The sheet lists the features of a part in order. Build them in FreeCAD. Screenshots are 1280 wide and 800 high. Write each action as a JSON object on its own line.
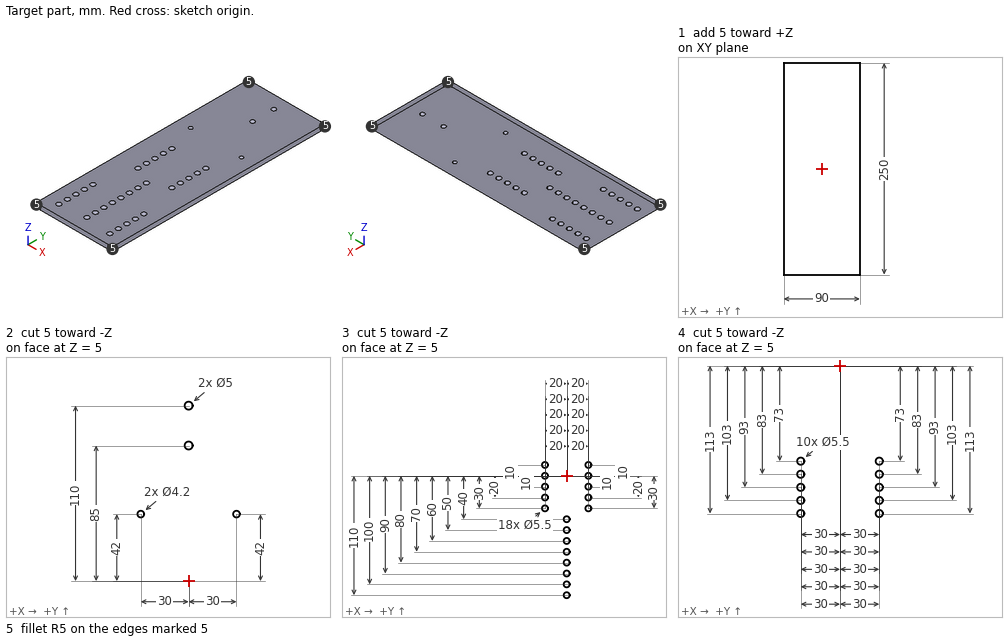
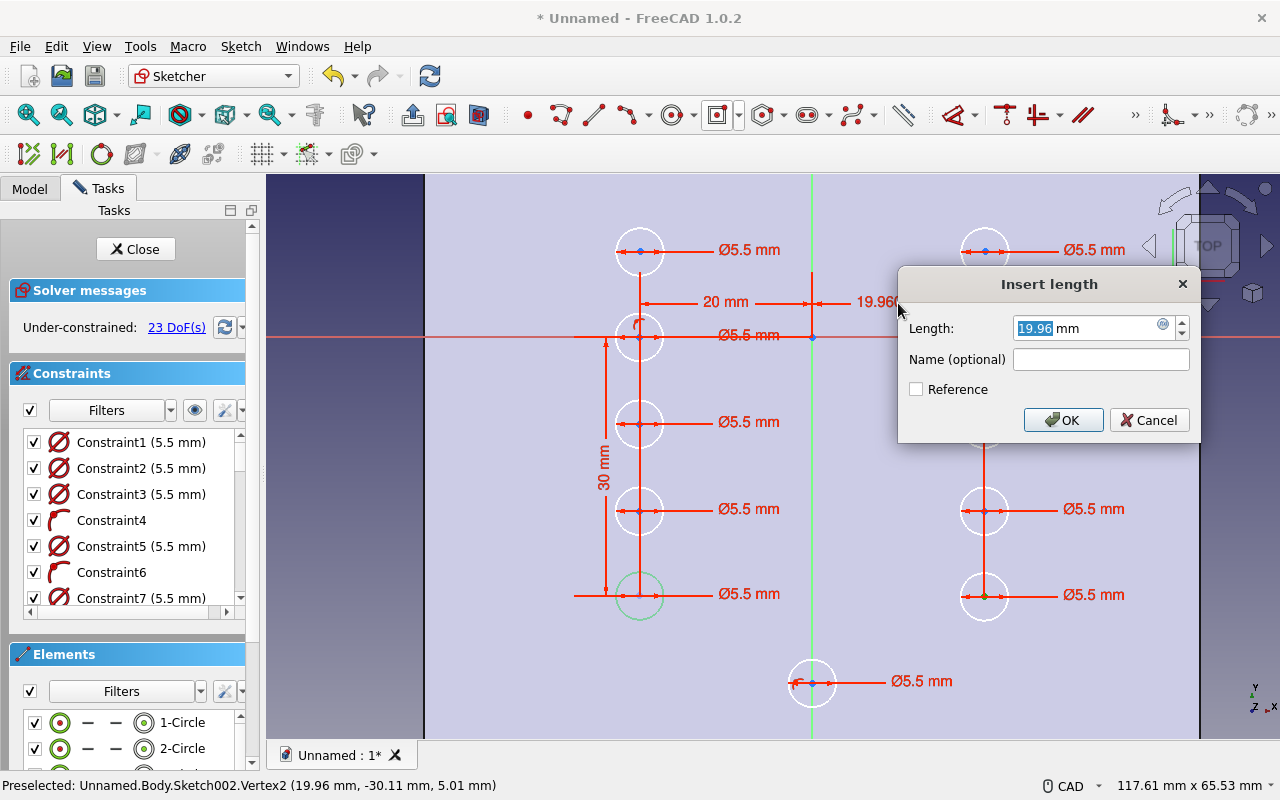
{"action": "type", "text": "20"}
{"action": "key", "text": "Return"}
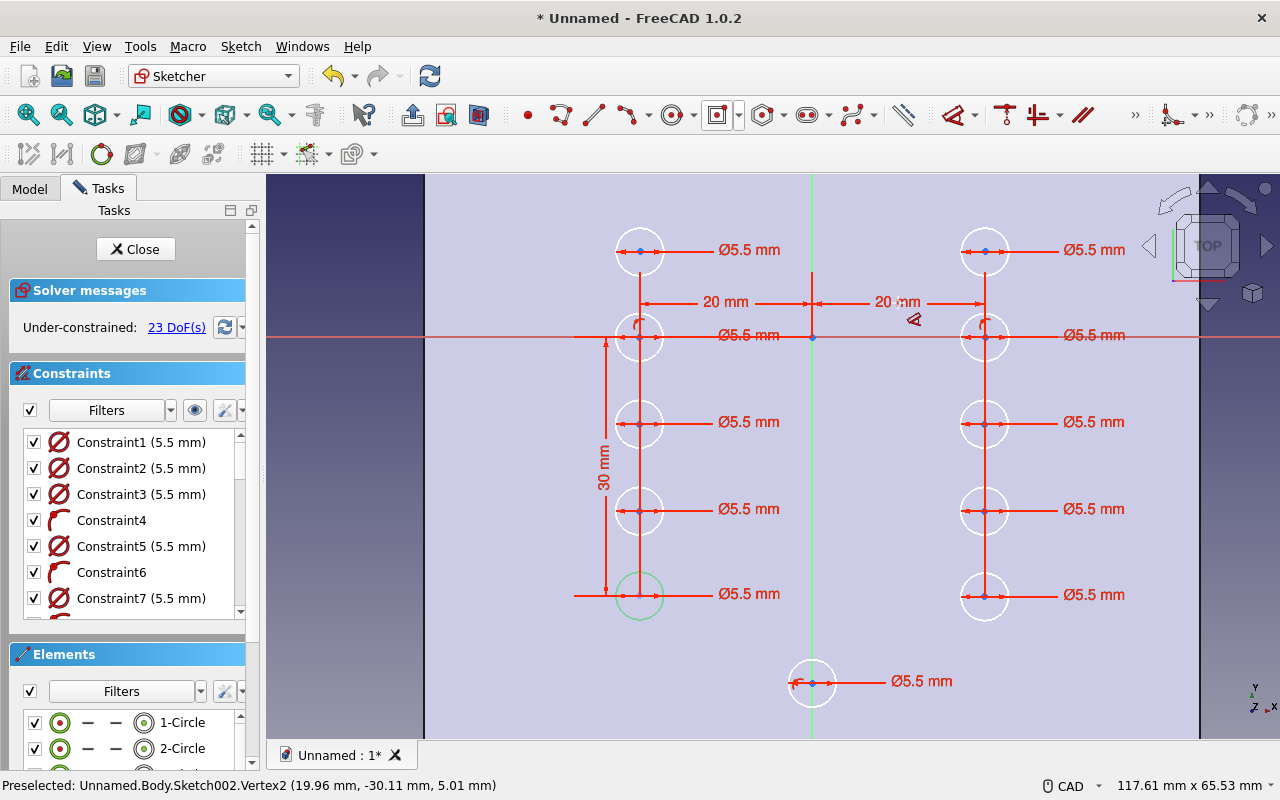
{"action": "left_click", "coordinate": [985, 597]}
{"action": "left_click", "coordinate": [1019, 467]}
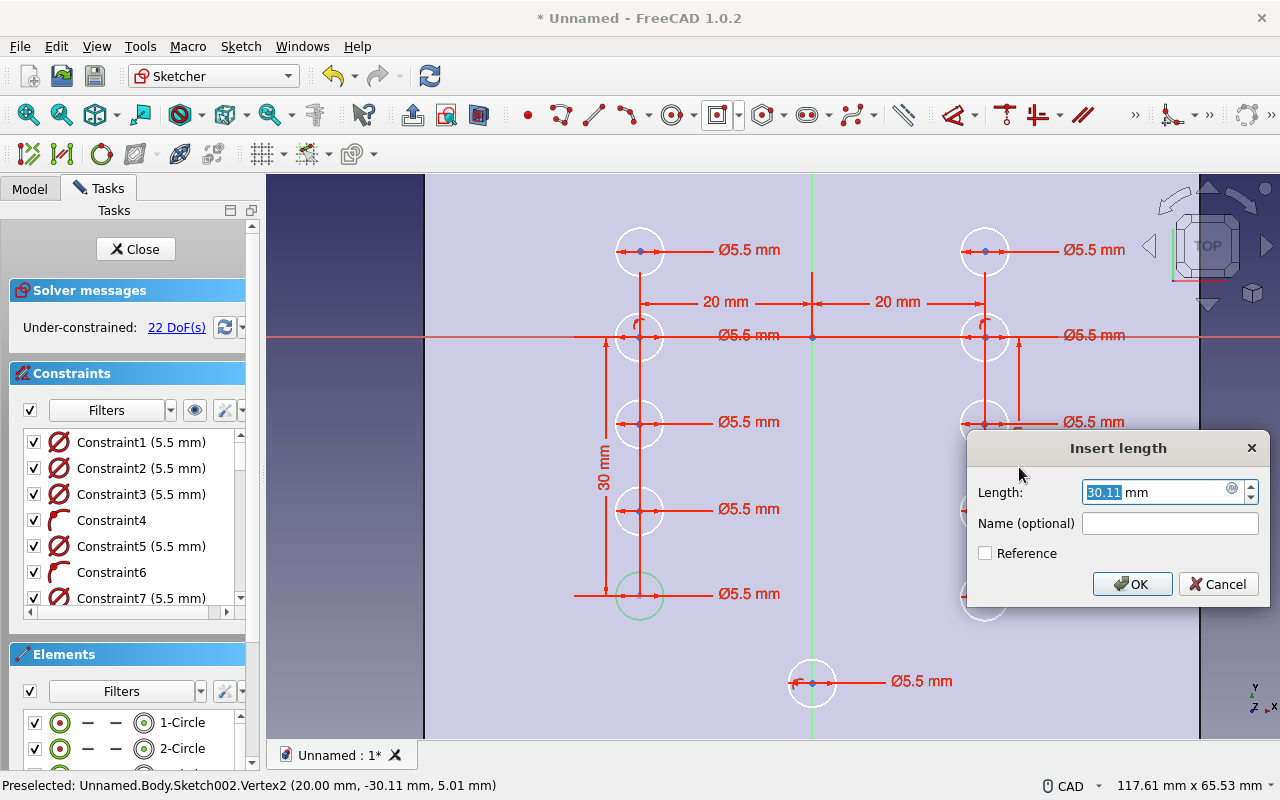
{"action": "type", "text": "30"}
{"action": "key", "text": "Return"}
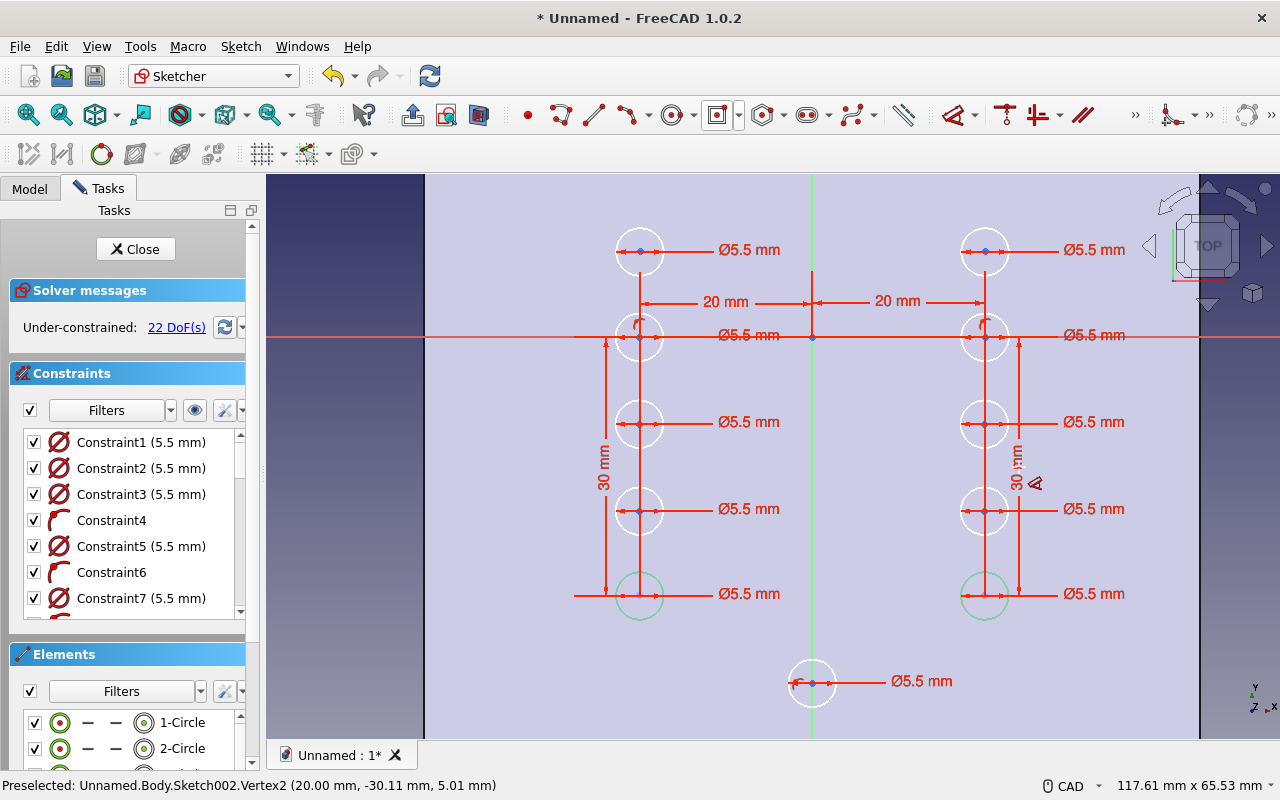
{"action": "scroll", "coordinate": [658, 322], "scroll_direction": "down", "scroll_amount": 6}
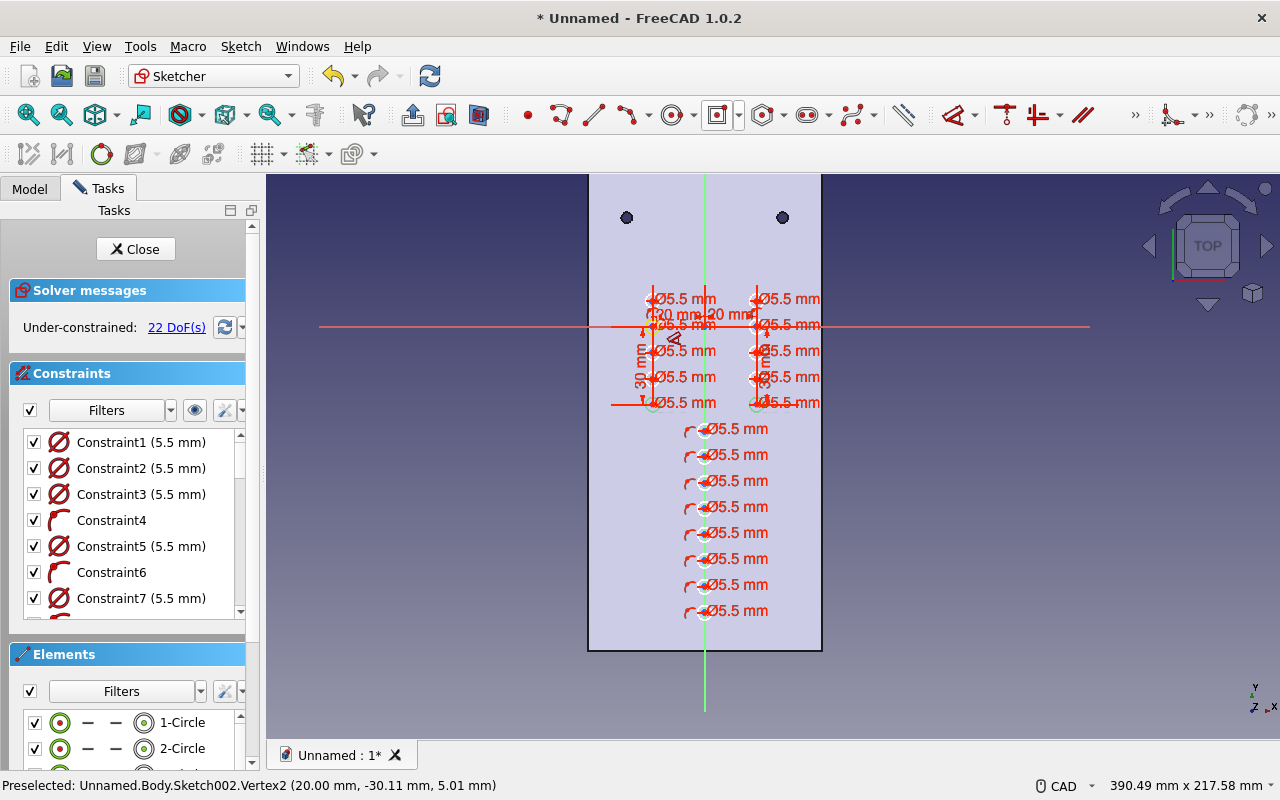
{"action": "left_click", "coordinate": [705, 535]}
{"action": "left_click", "coordinate": [739, 431]}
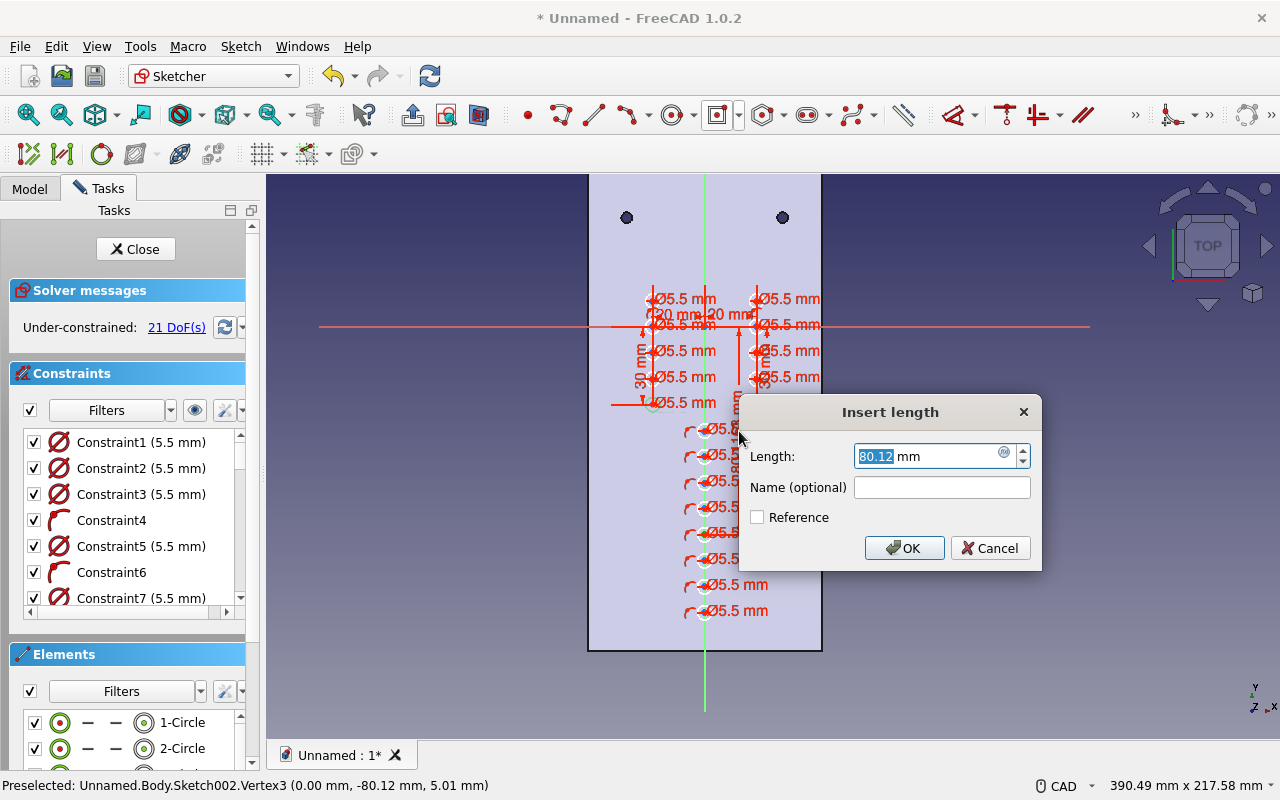
{"action": "type", "text": "80"}
{"action": "key", "text": "Return"}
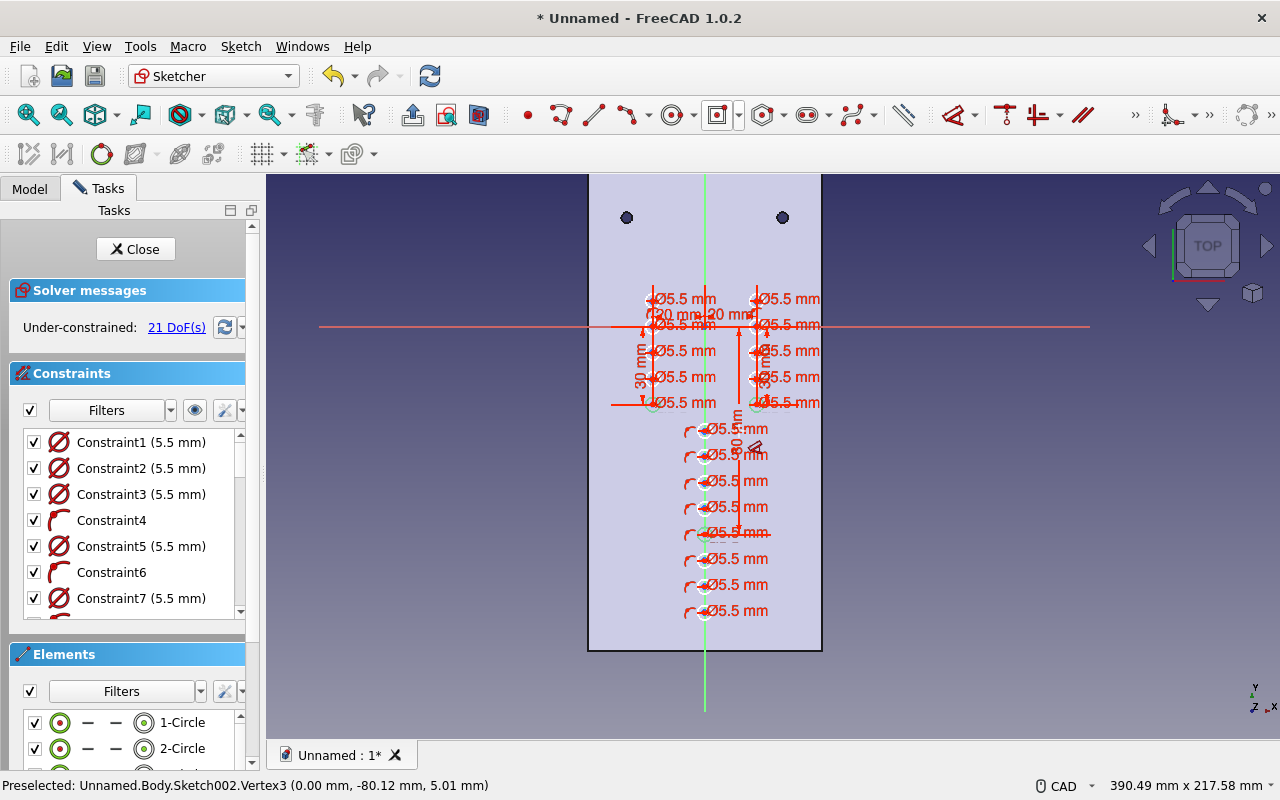
{"action": "left_click", "coordinate": [705, 509]}
{"action": "left_click", "coordinate": [739, 460]}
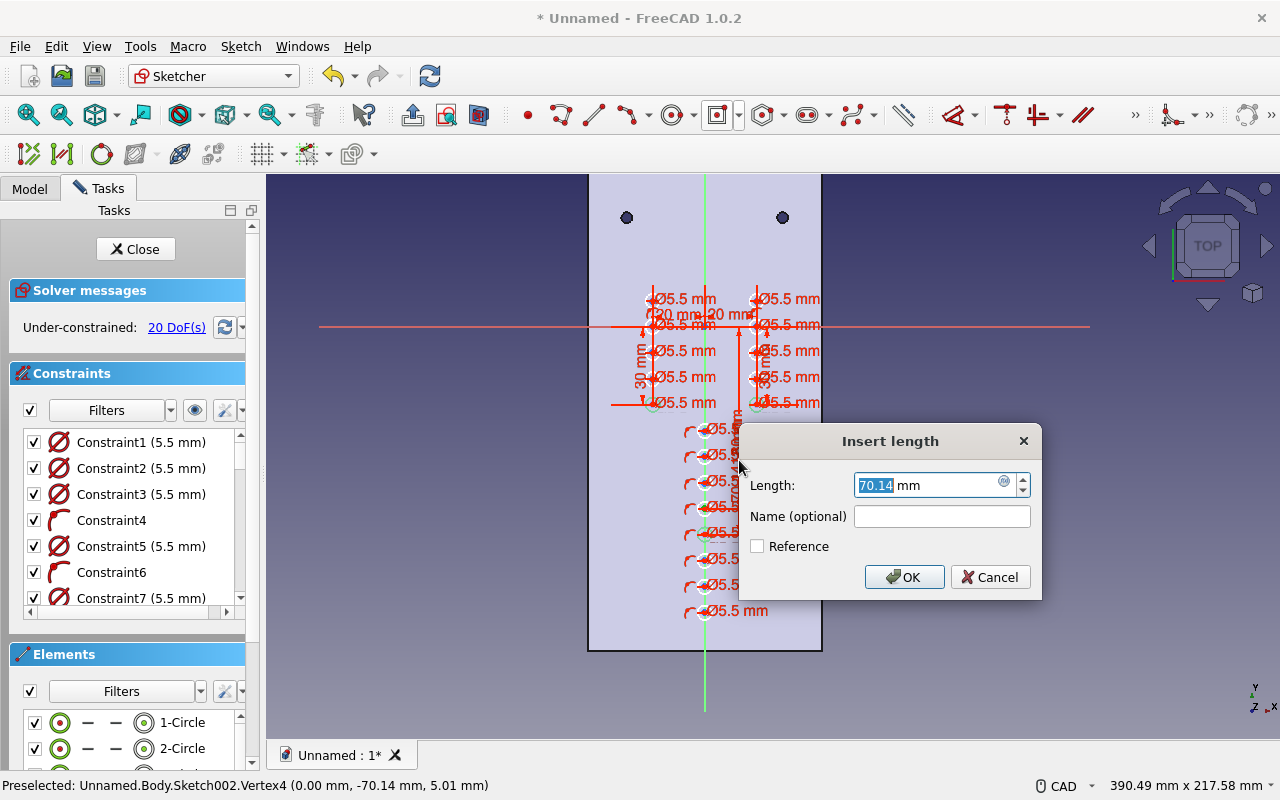
{"action": "type", "text": "70"}
{"action": "key", "text": "Return"}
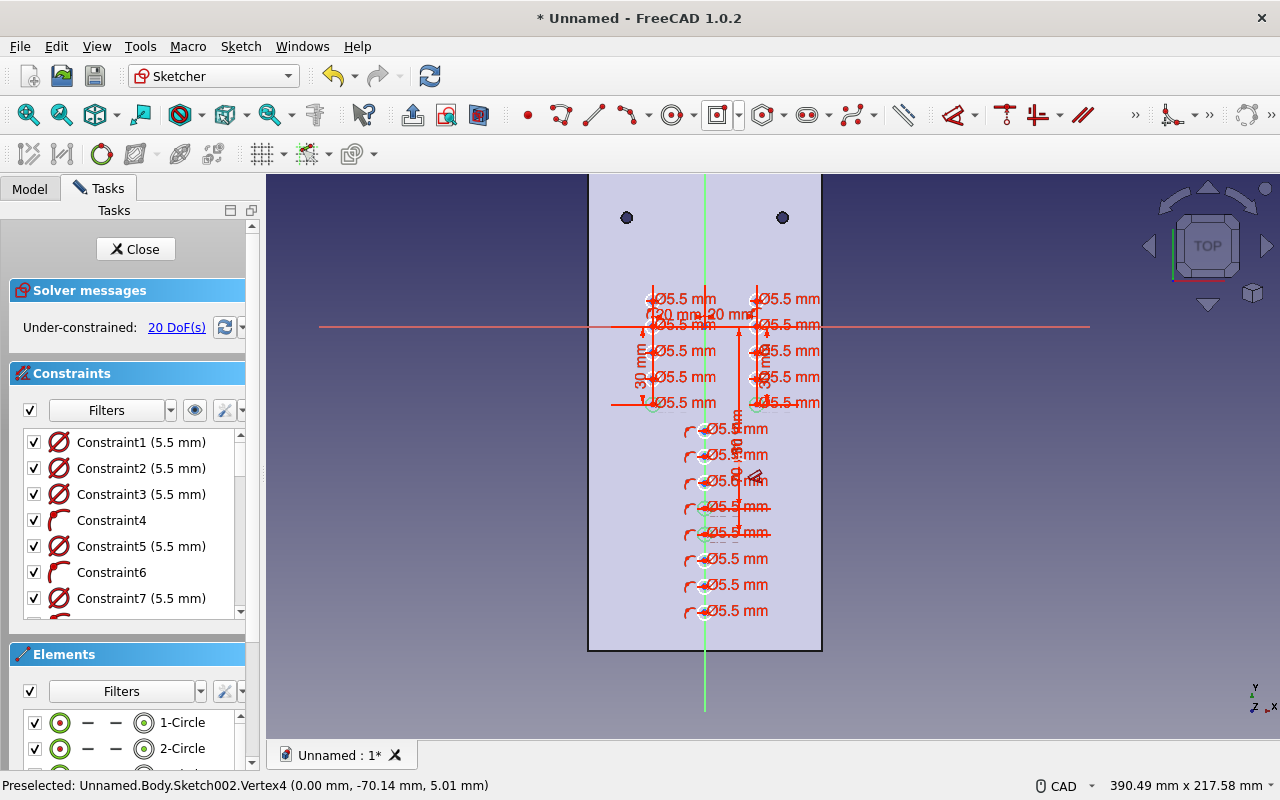
{"action": "left_click", "coordinate": [705, 483]}
{"action": "left_click", "coordinate": [647, 441]}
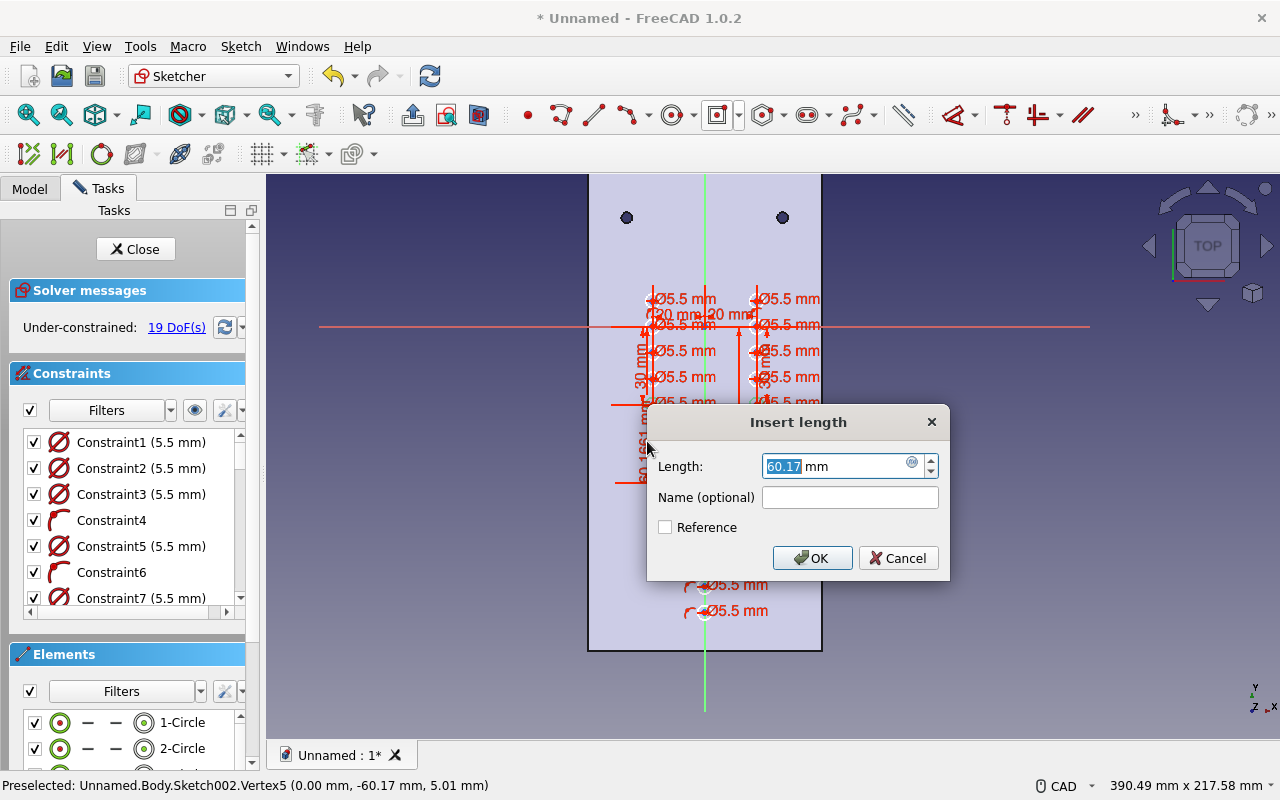
{"action": "type", "text": "60"}
{"action": "key", "text": "Return"}